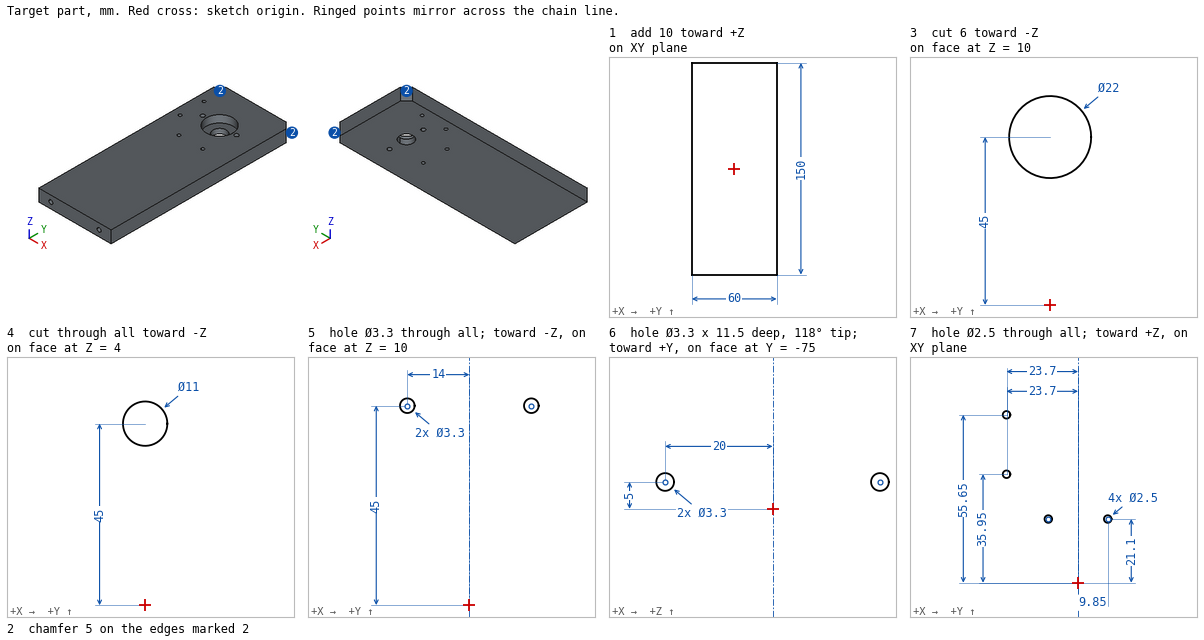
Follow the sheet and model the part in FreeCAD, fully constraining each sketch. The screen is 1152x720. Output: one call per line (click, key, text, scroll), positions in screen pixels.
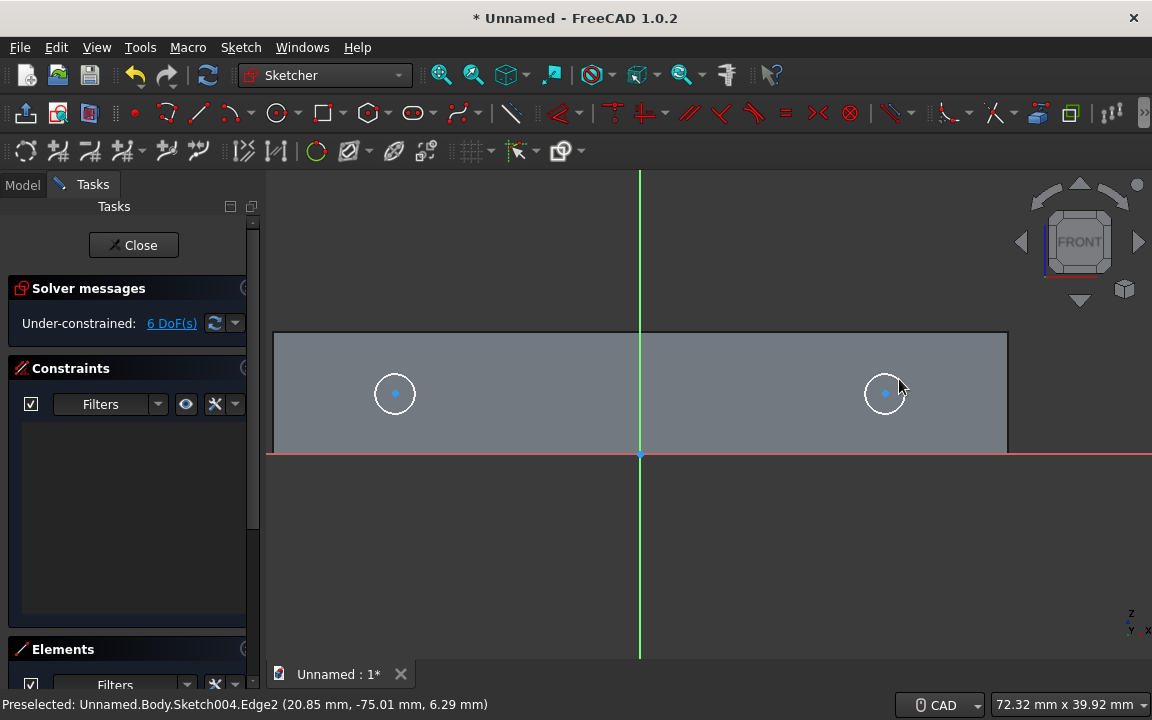
click(409, 380)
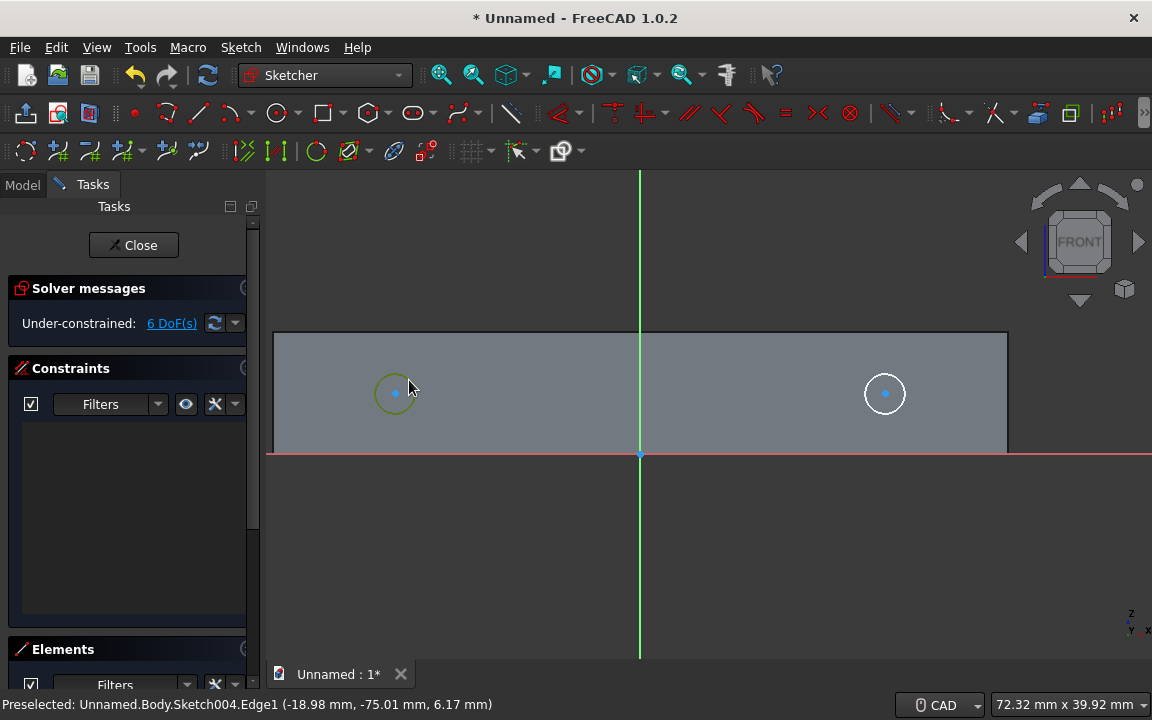
click(899, 380)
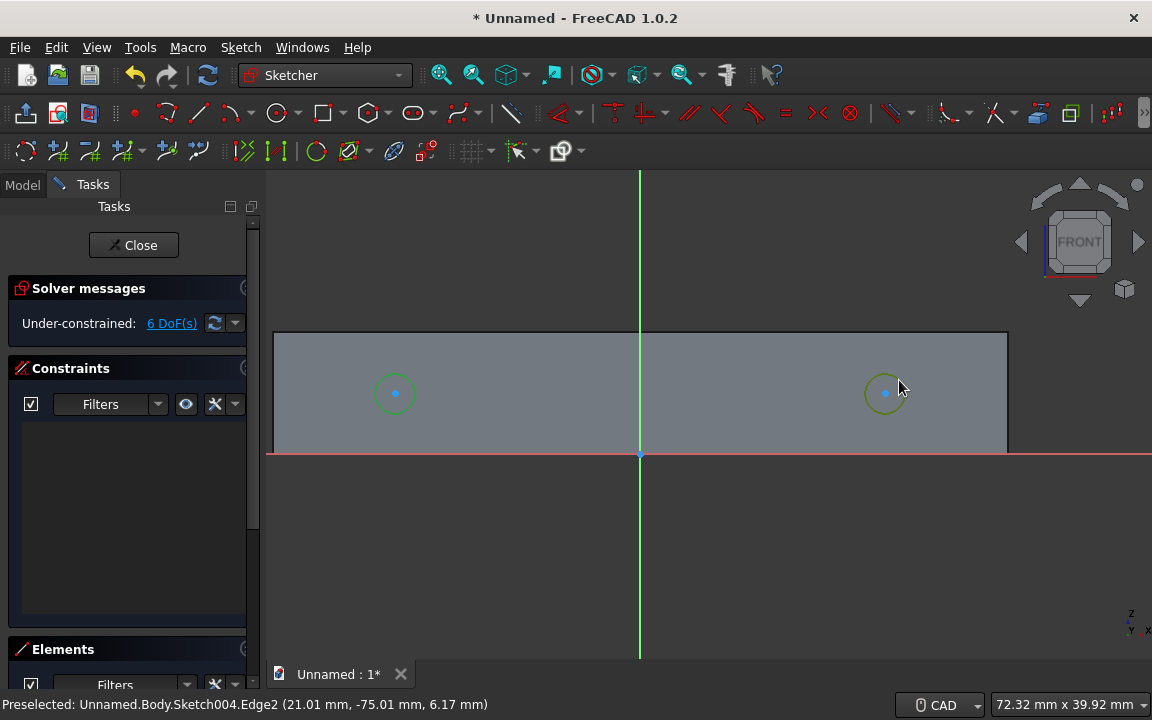
click(786, 114)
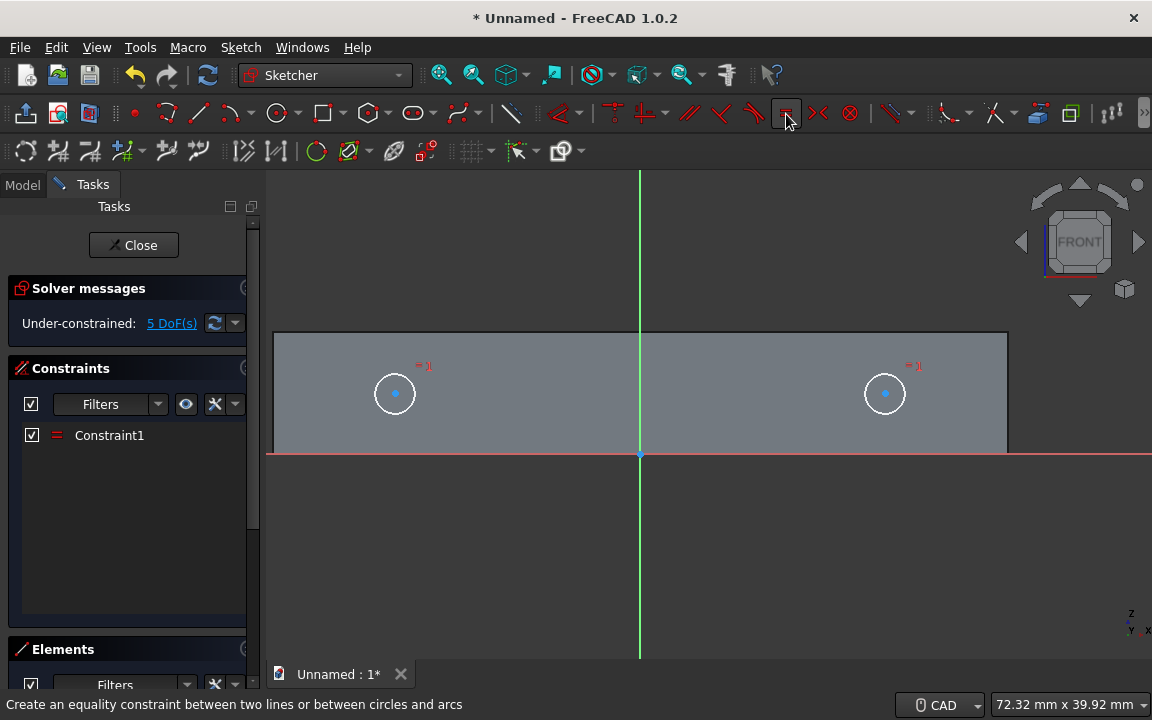
click(395, 394)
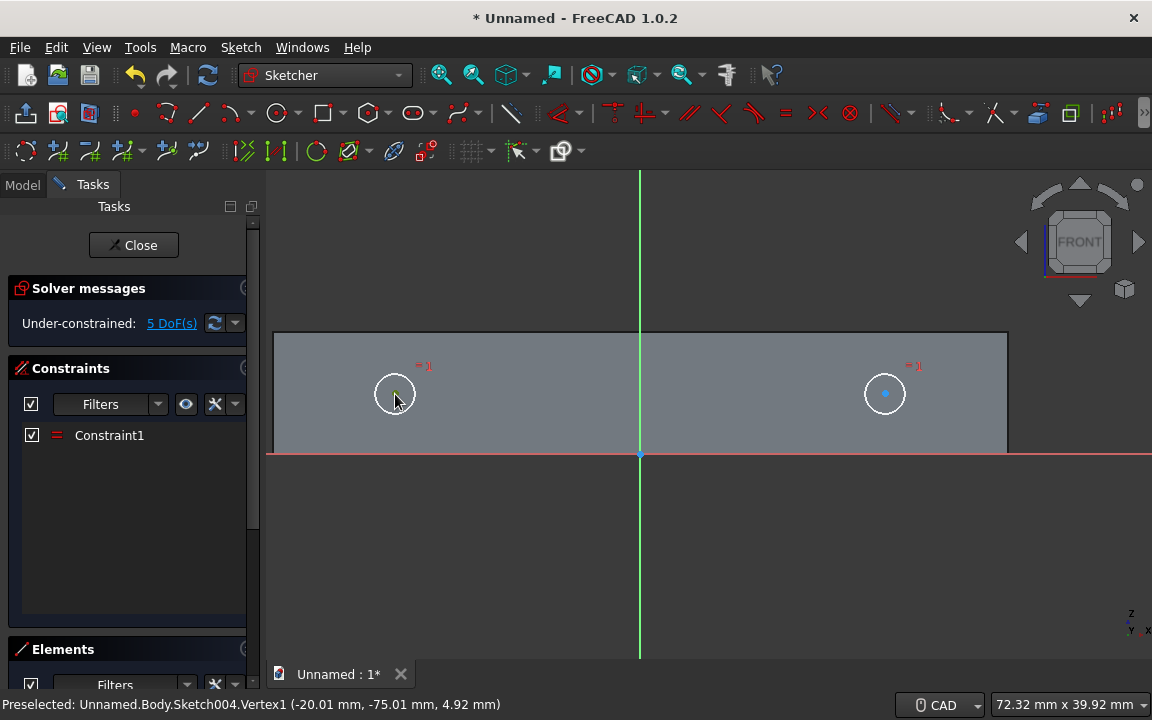
click(885, 394)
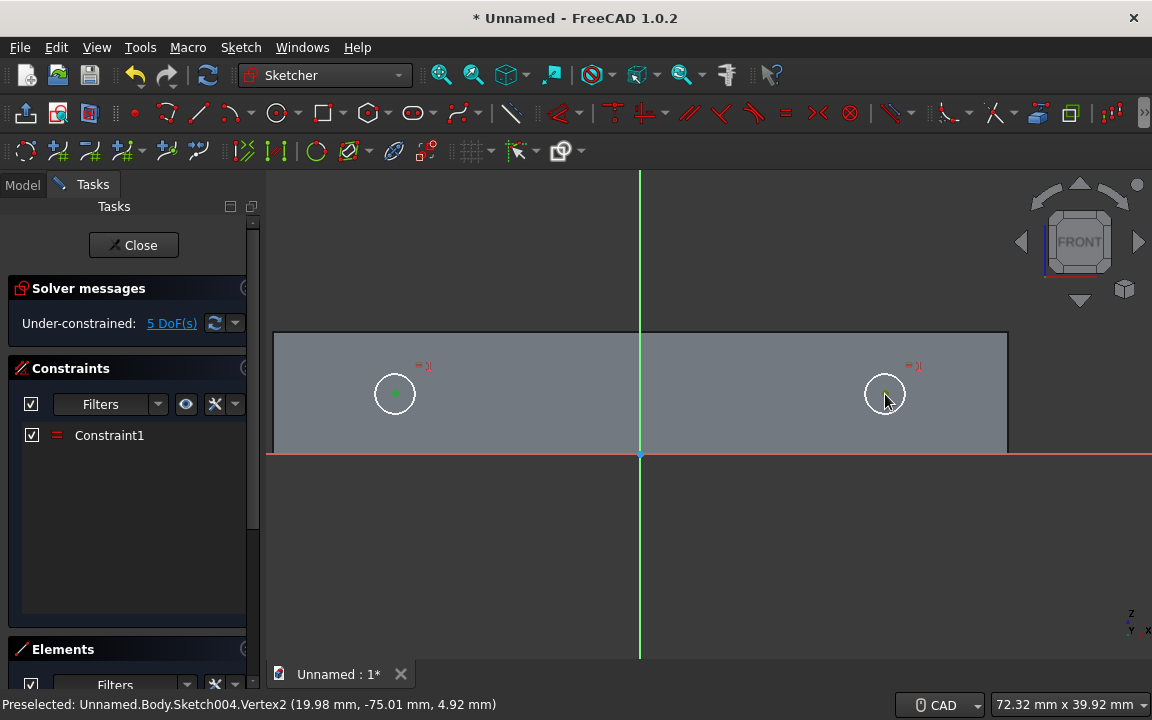
click(640, 600)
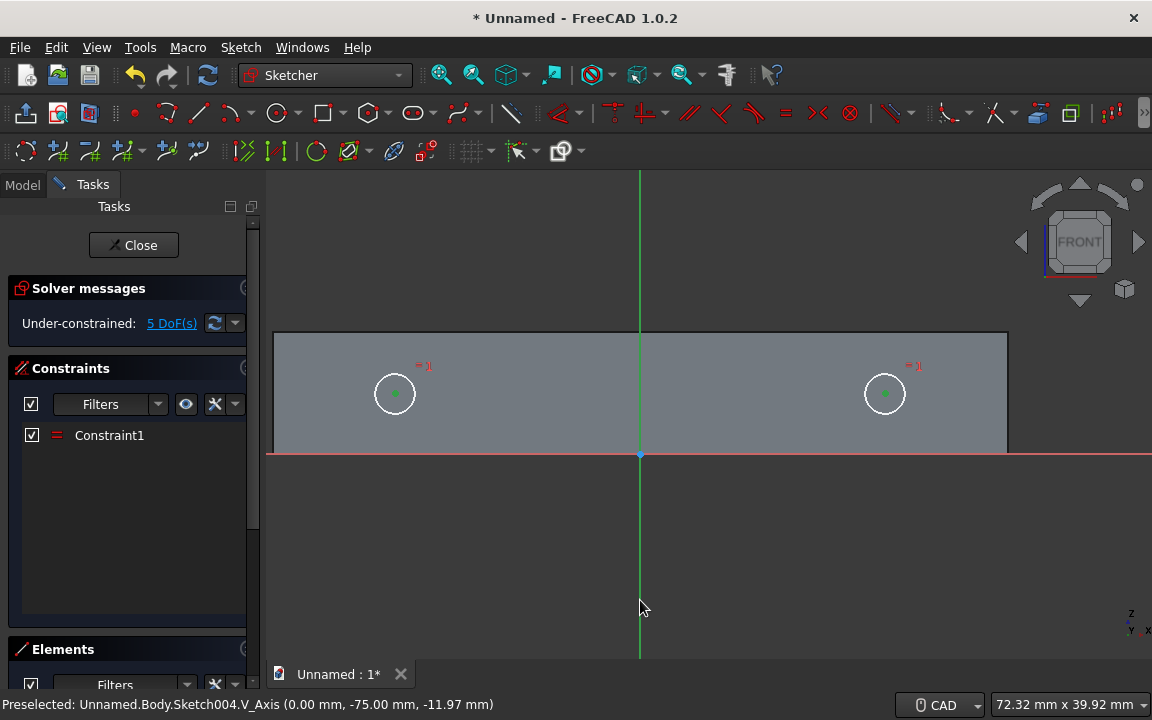
click(818, 114)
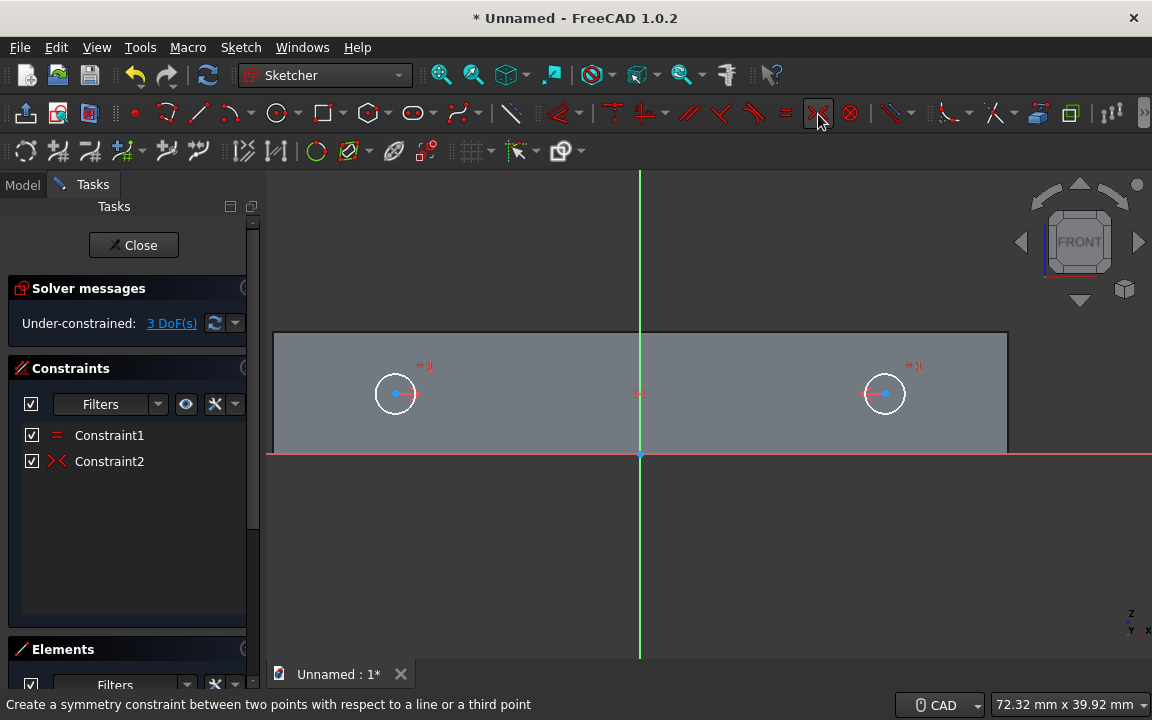
click(558, 114)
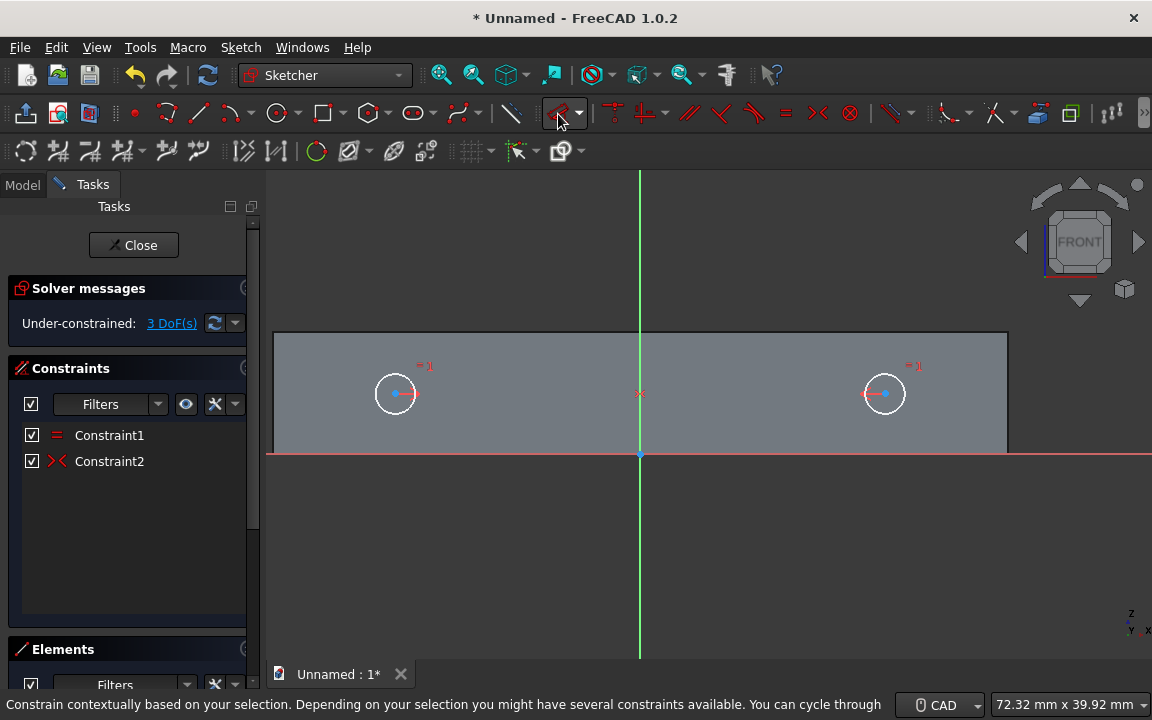
click(409, 380)
click(431, 357)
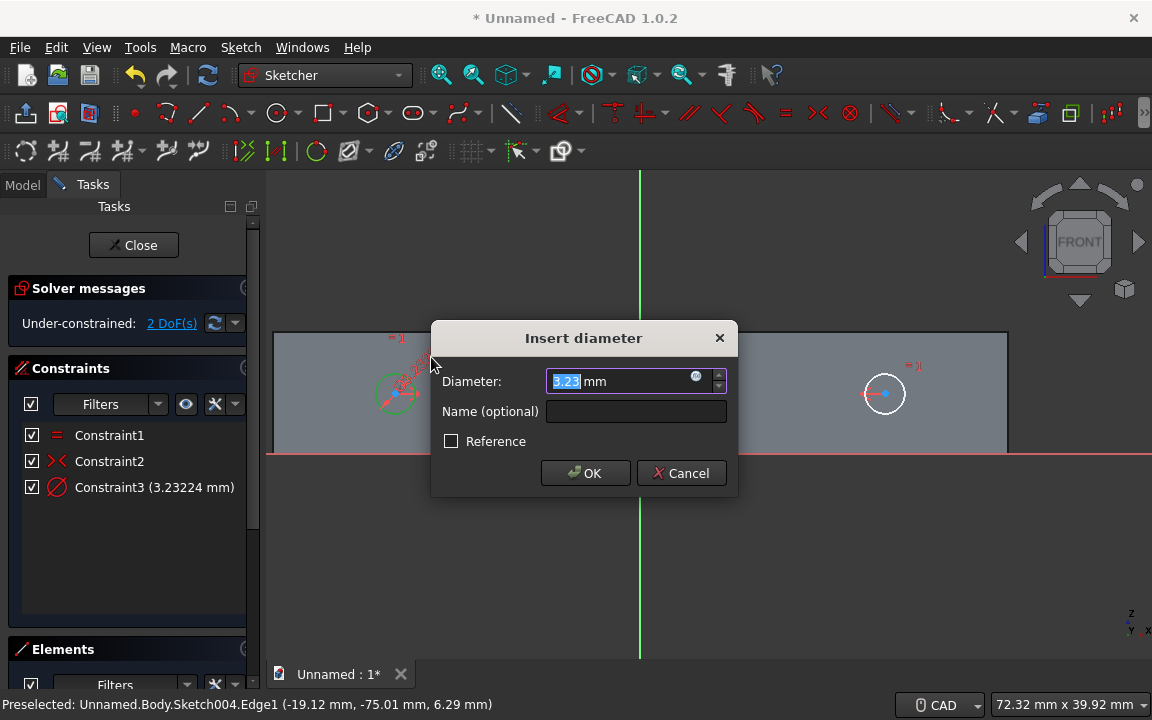
text(3.3)
key(Return)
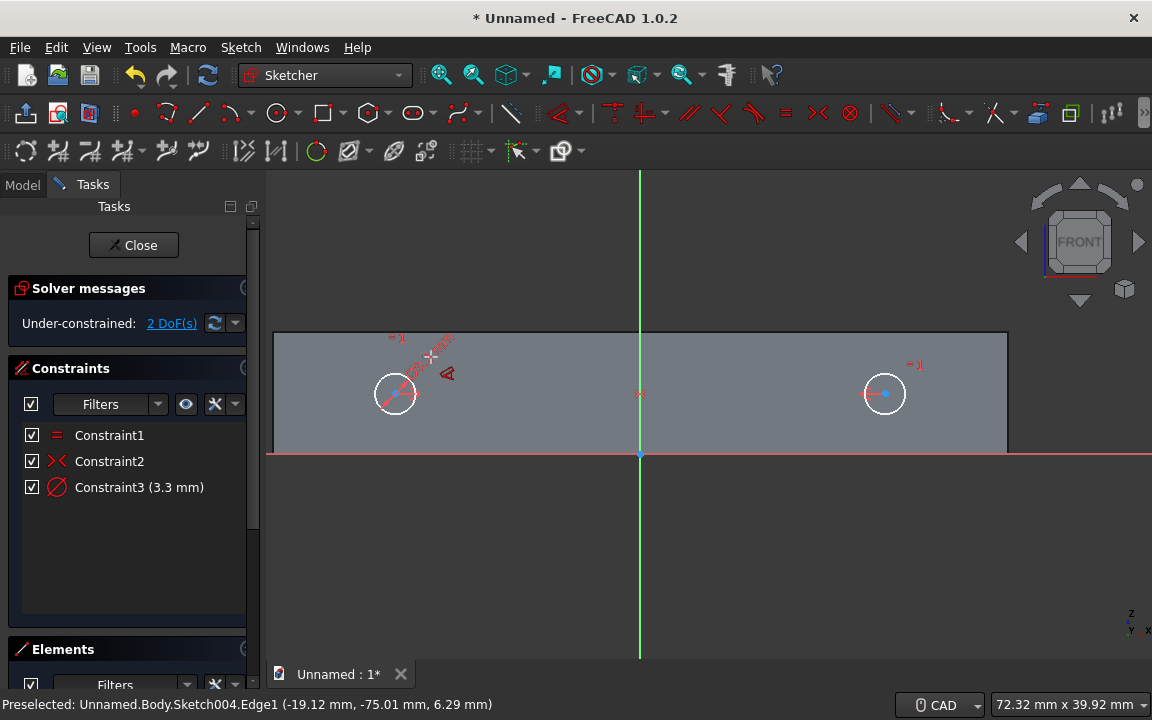
click(395, 394)
click(361, 424)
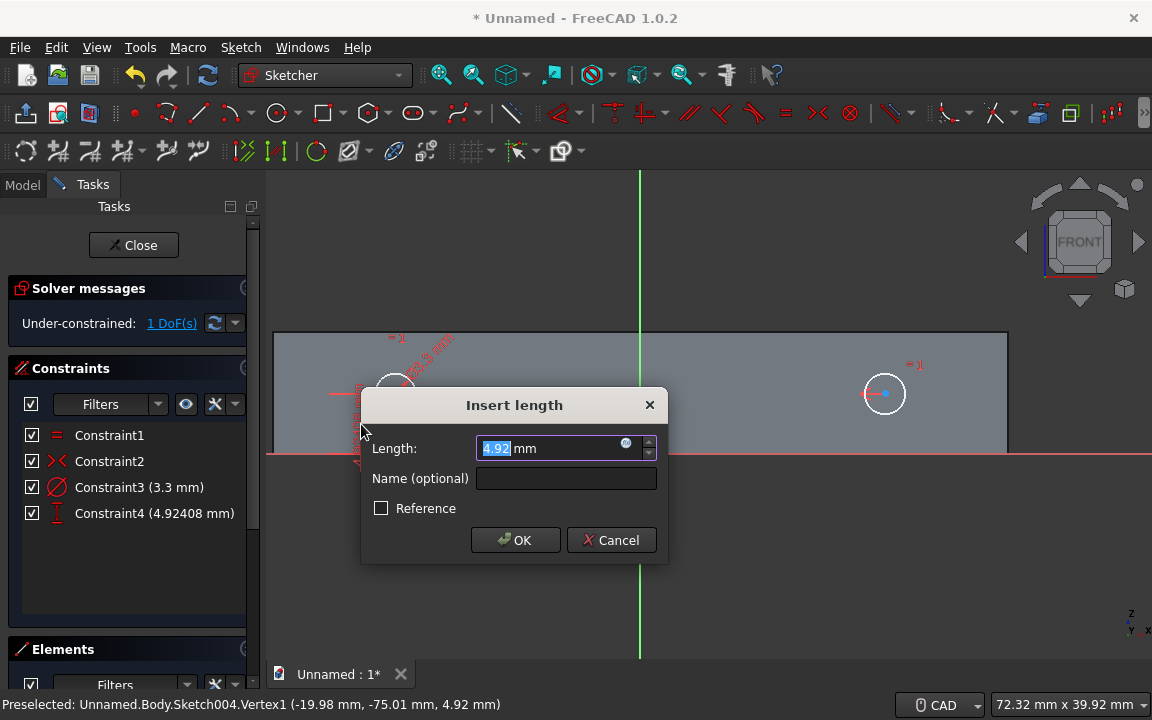
text(5)
key(Return)